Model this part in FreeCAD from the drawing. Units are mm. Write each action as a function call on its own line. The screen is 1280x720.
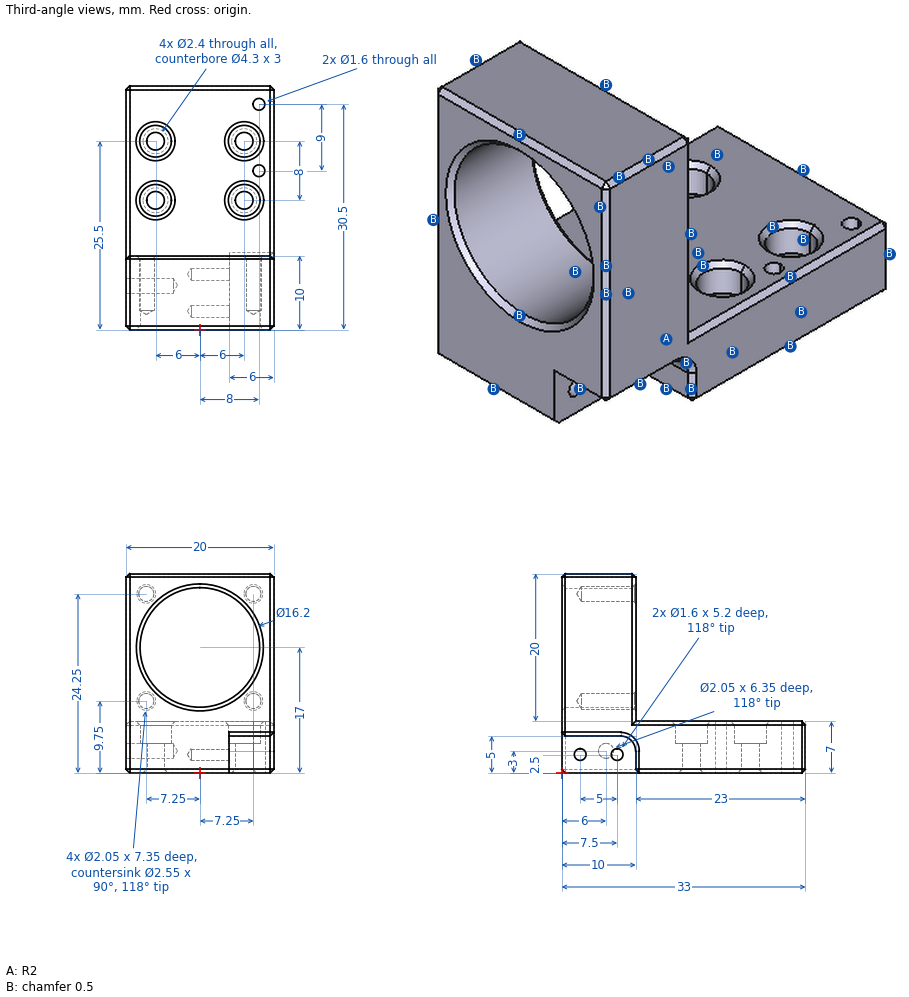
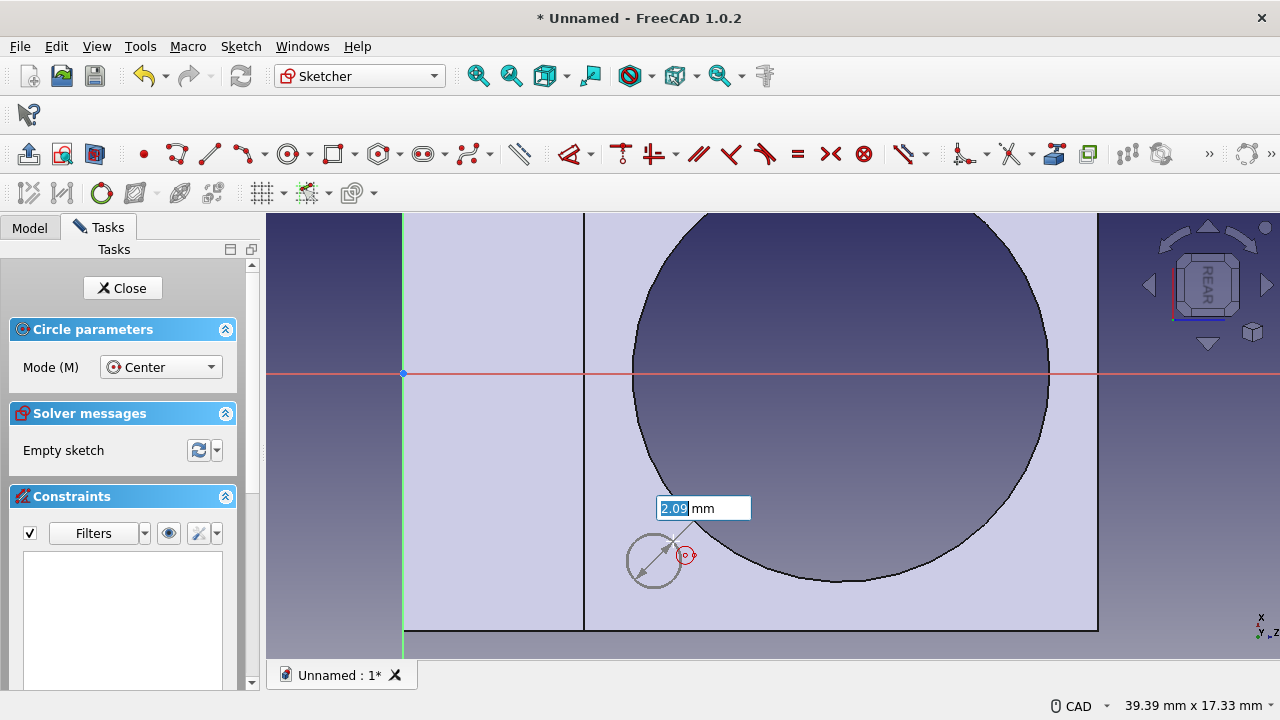
text(2.05)
key(Return)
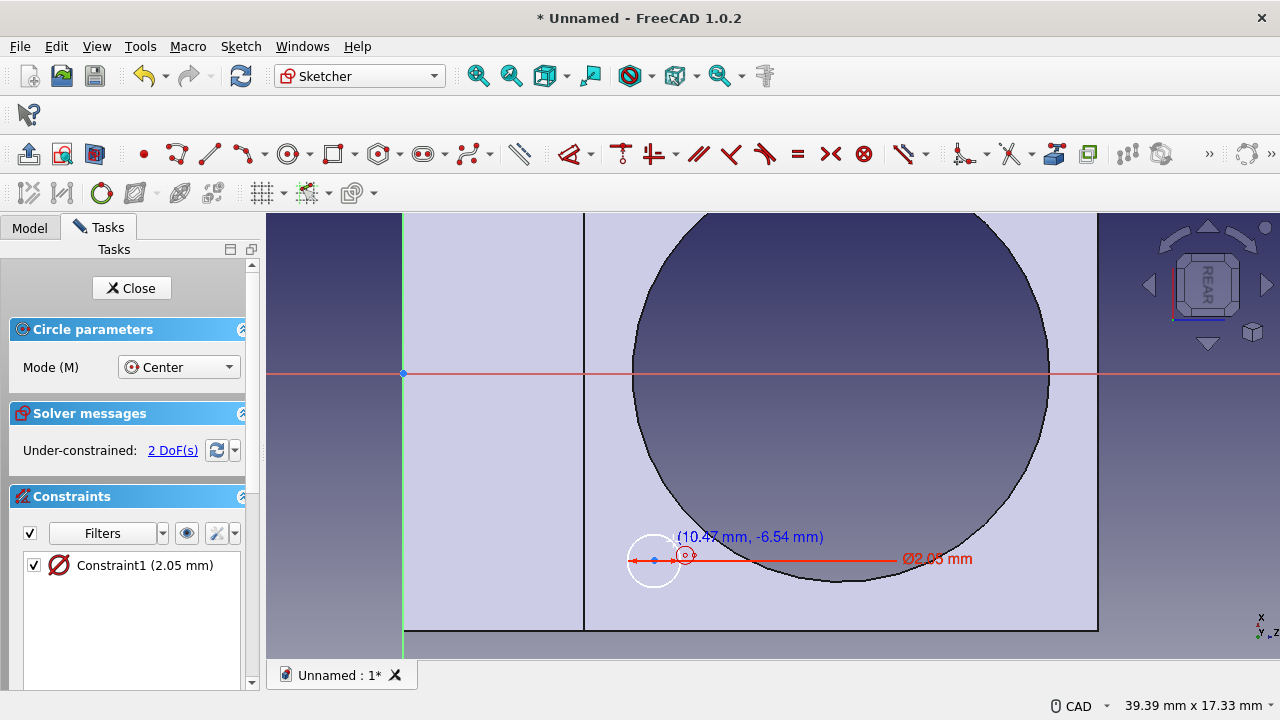
click(1028, 560)
move(1046, 541)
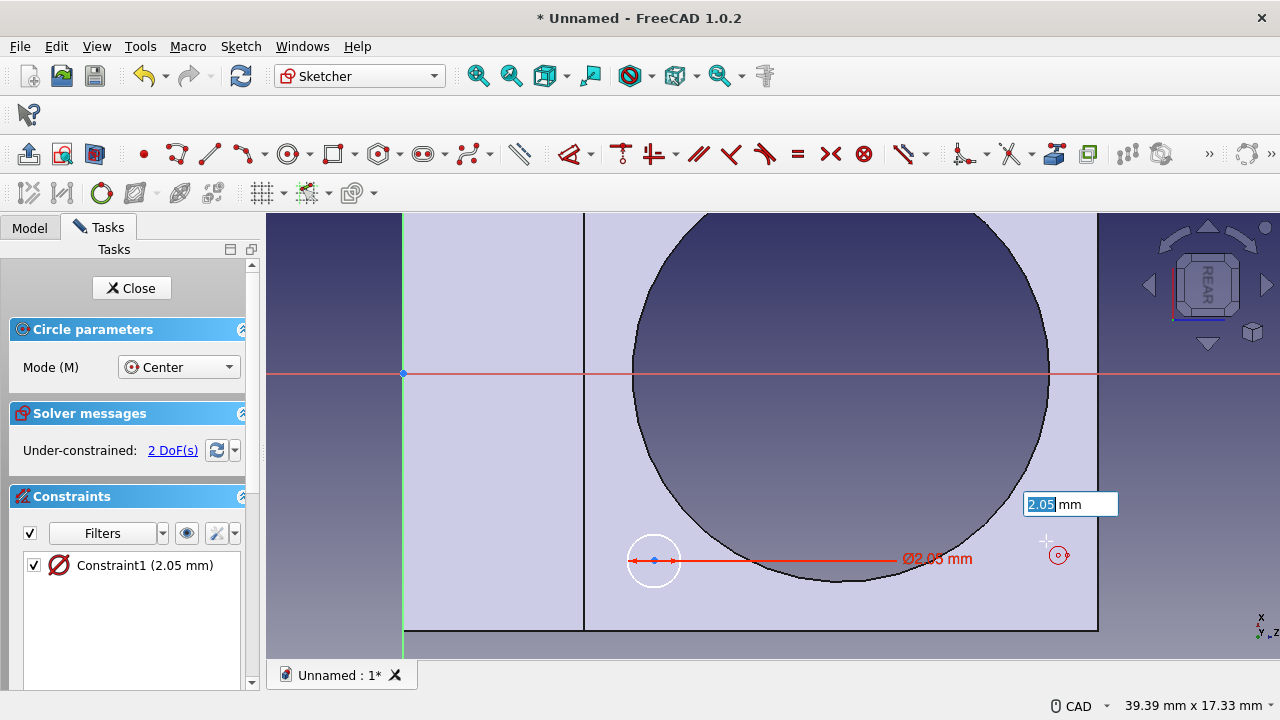
text(2.05)
key(Return)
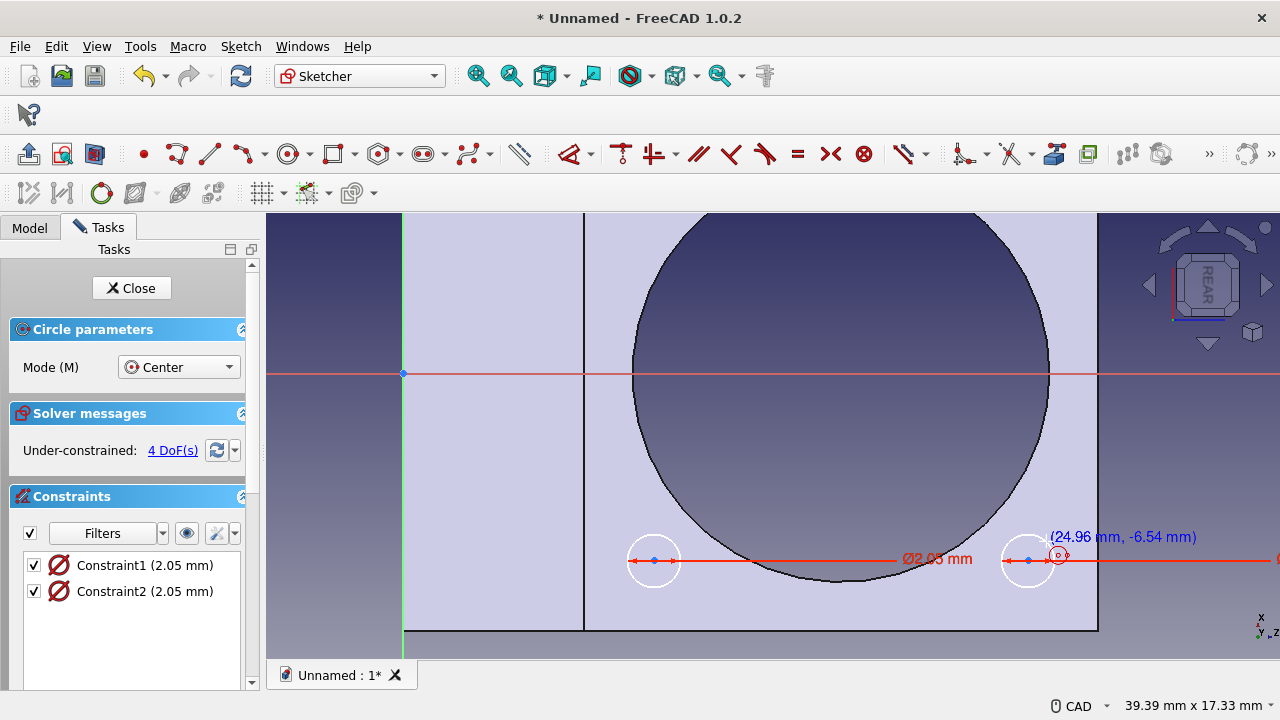
scroll(655, 563, down, 2)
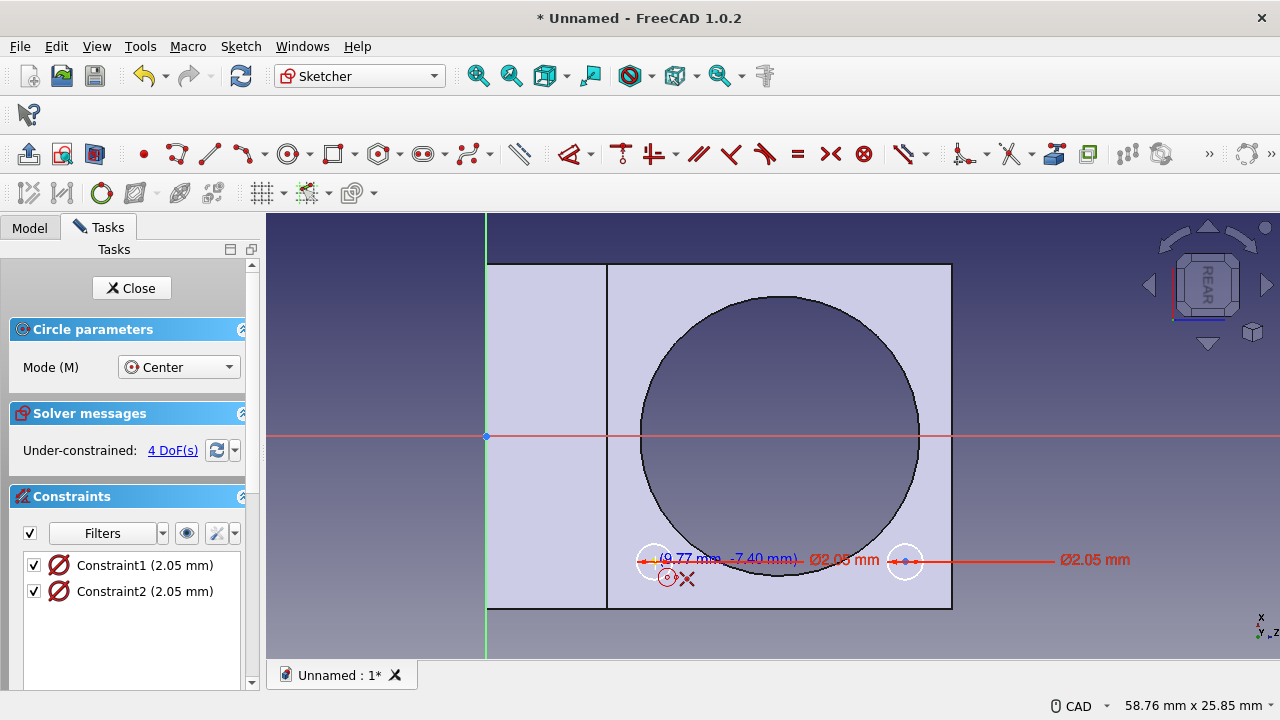
scroll(905, 311, up, 2)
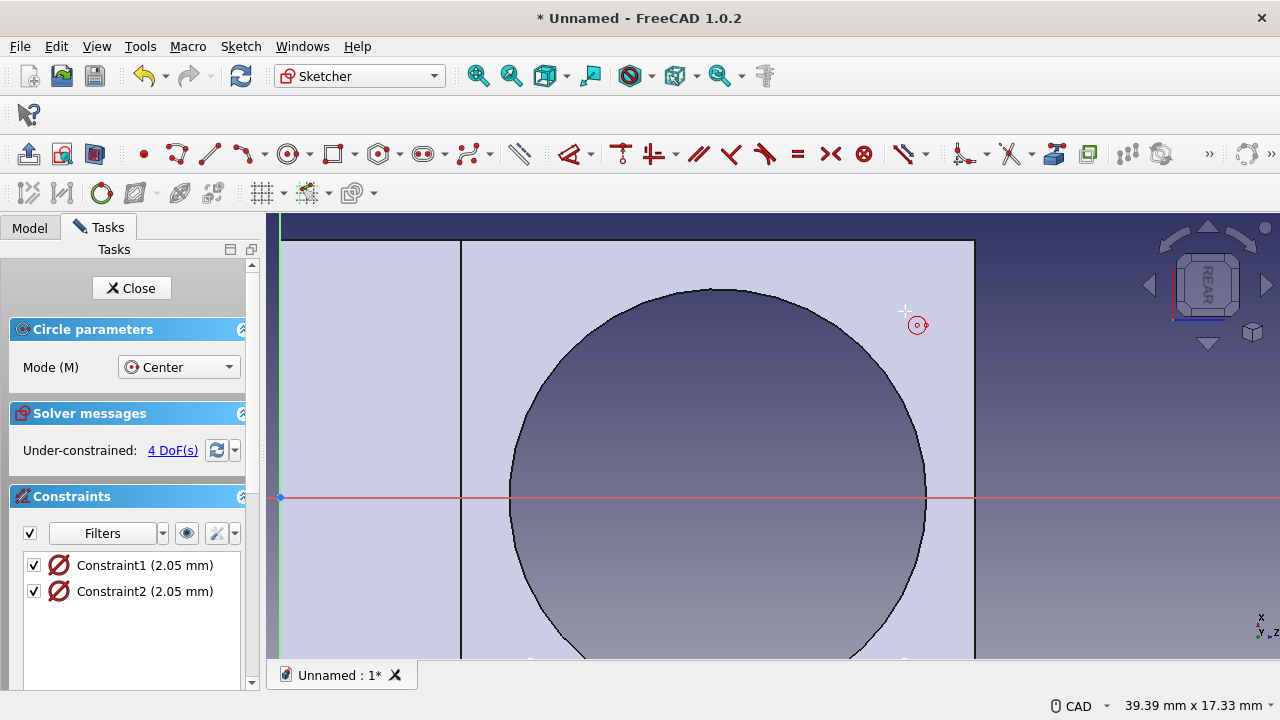
click(905, 311)
move(923, 292)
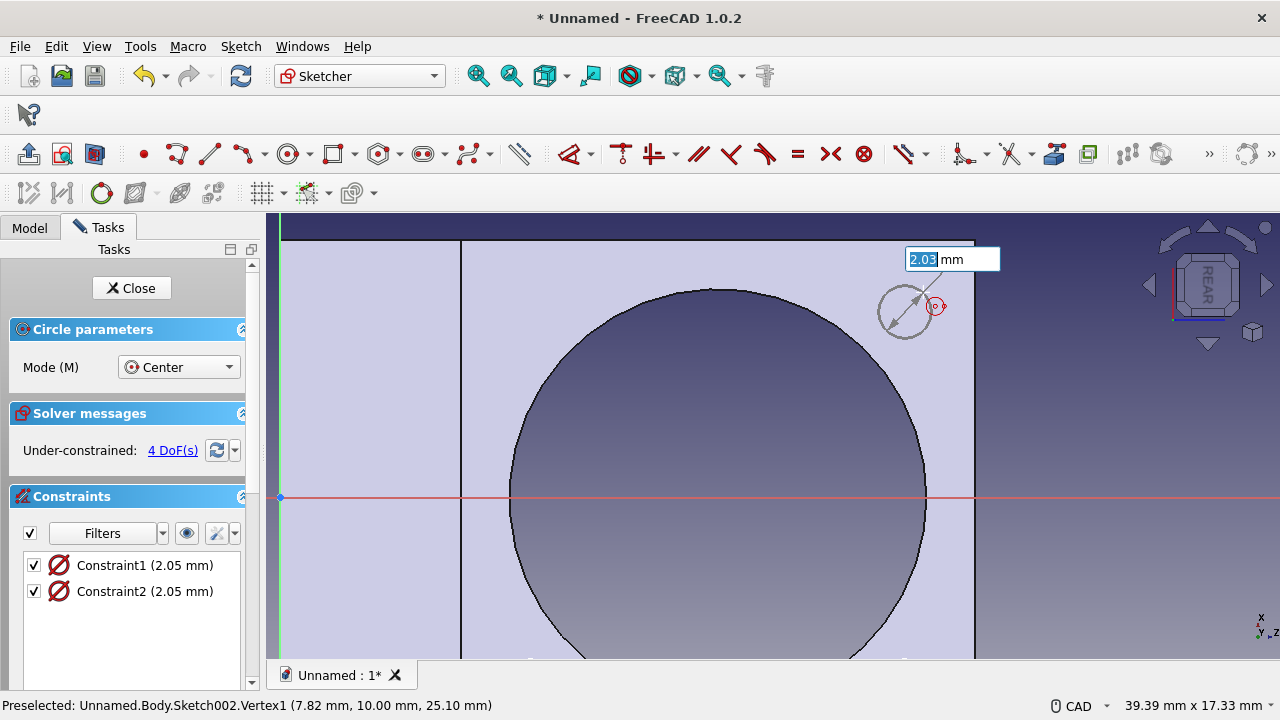
text(2.05)
key(Return)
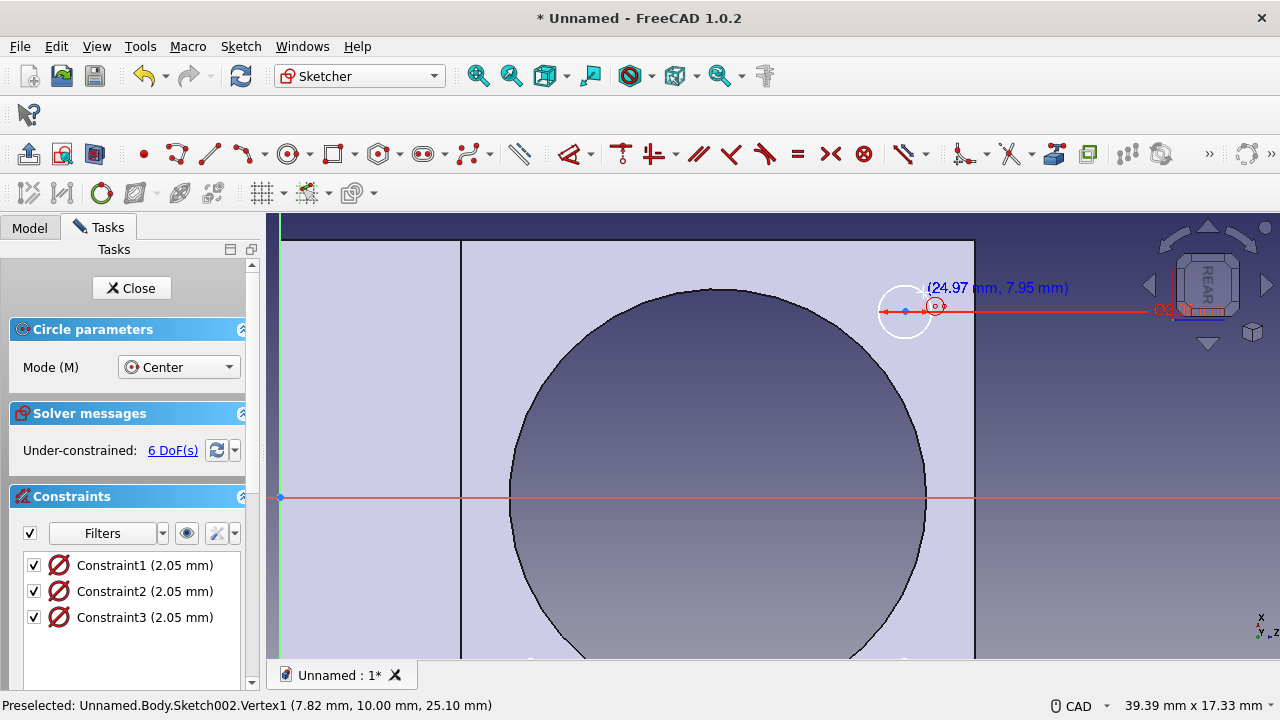
click(531, 311)
move(550, 292)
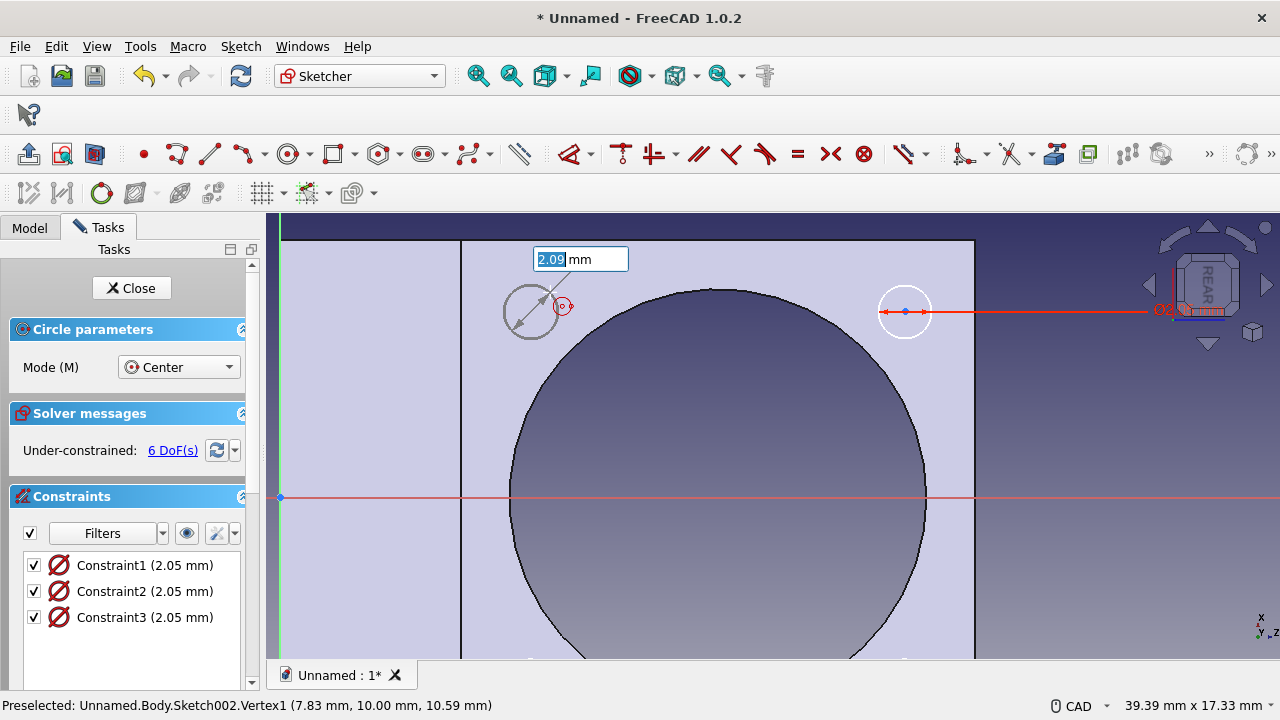
text(2.05)
key(Return)
key(Escape)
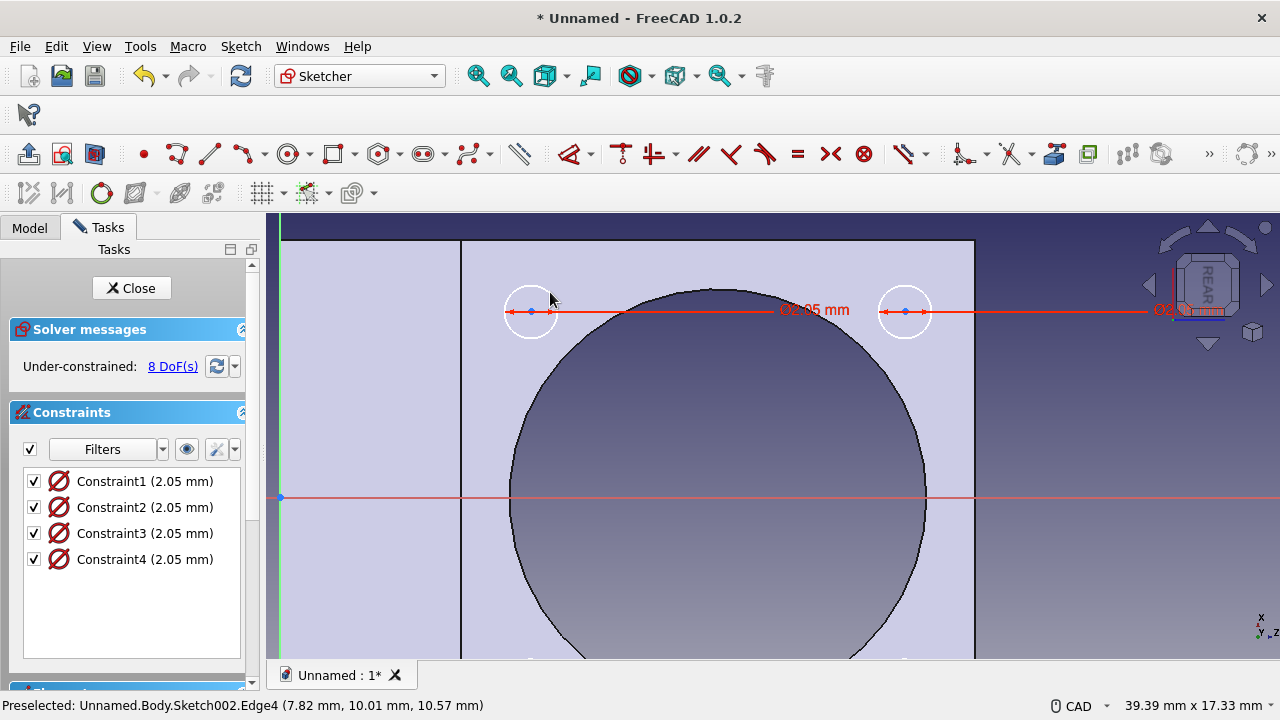
scroll(905, 310, down, 2)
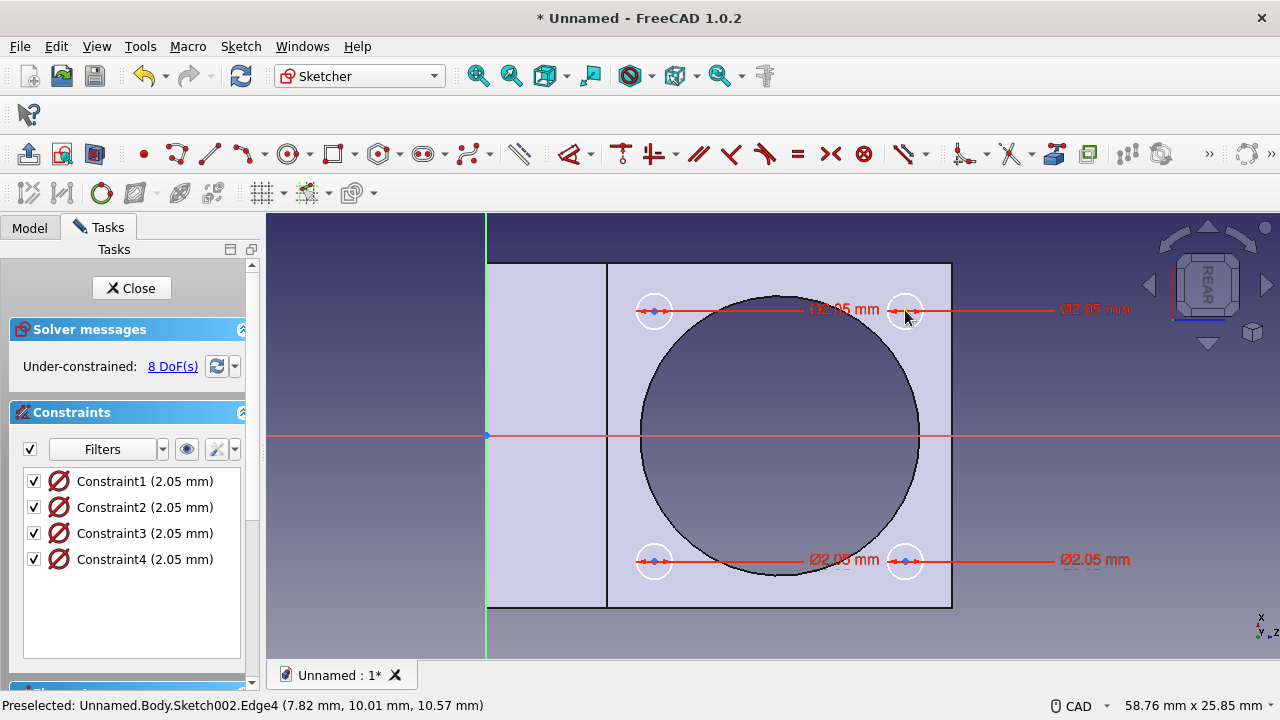
click(654, 562)